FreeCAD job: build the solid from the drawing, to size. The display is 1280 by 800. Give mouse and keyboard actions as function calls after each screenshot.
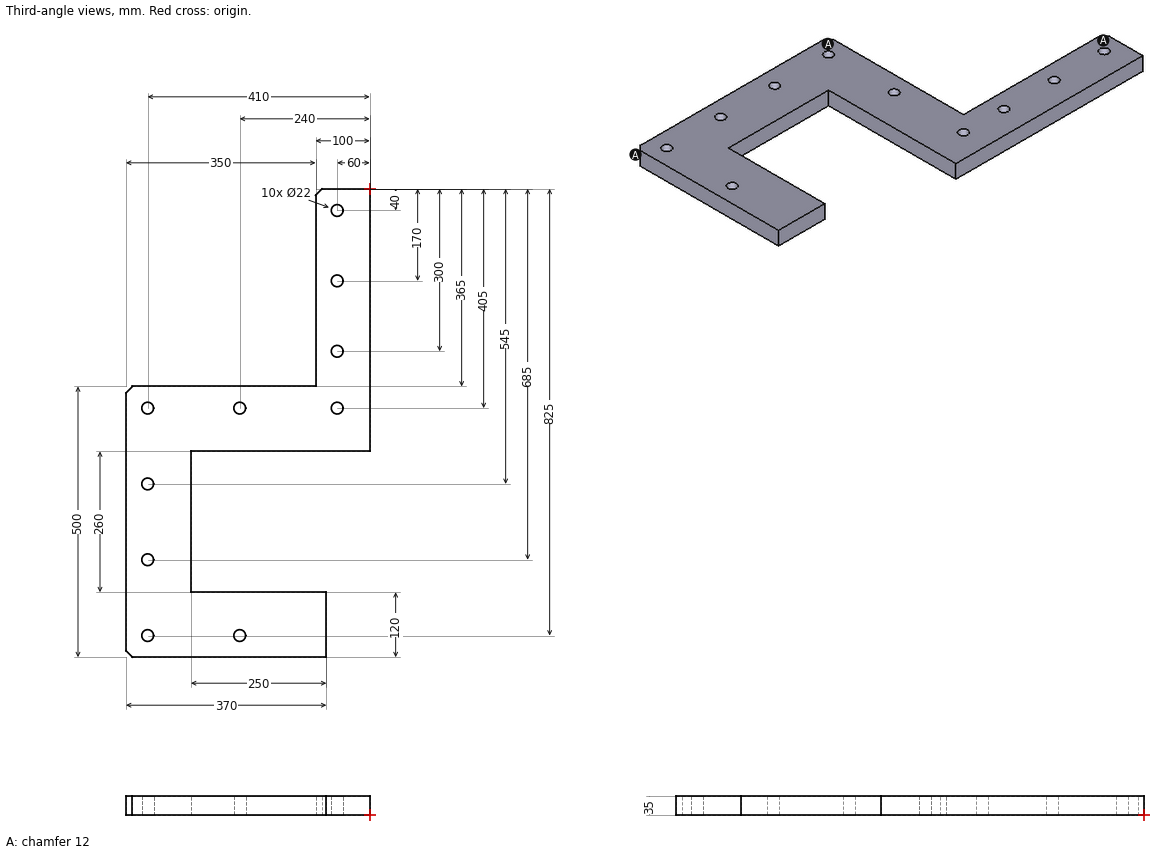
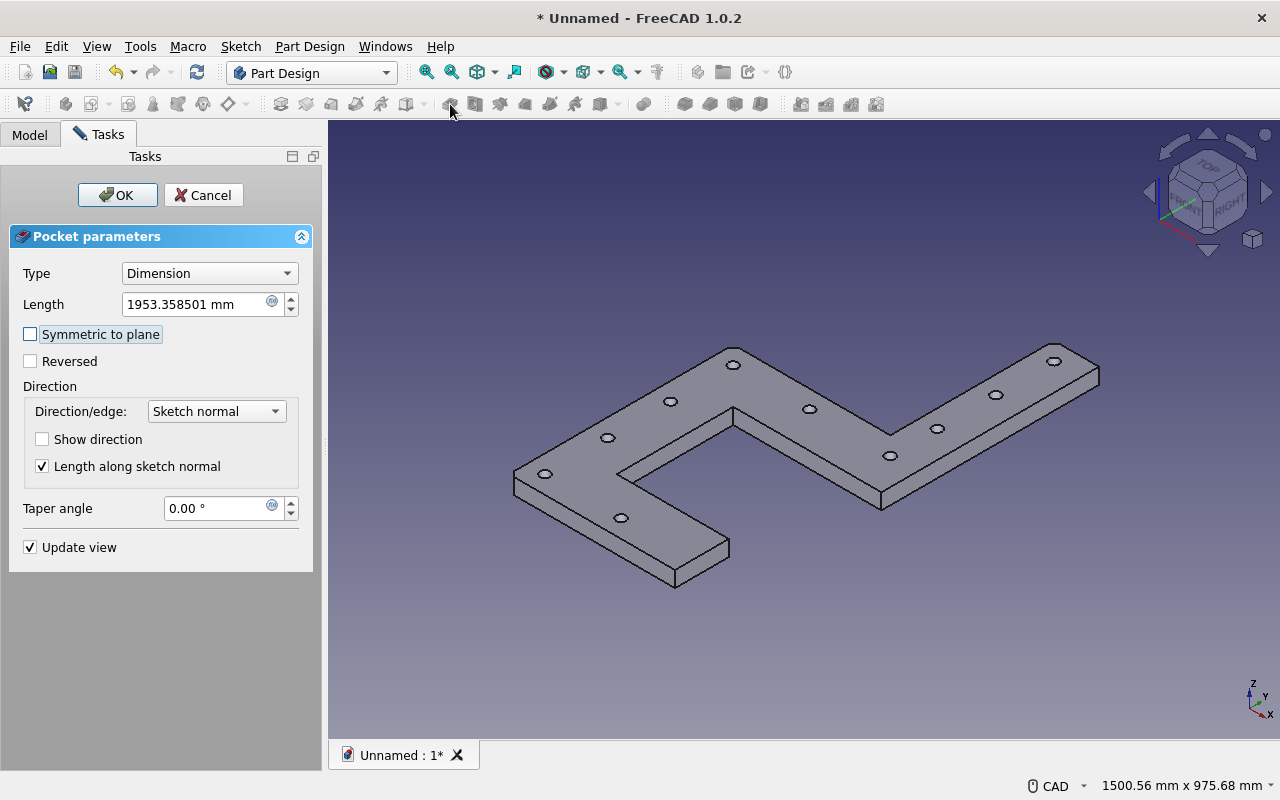
click(31, 334)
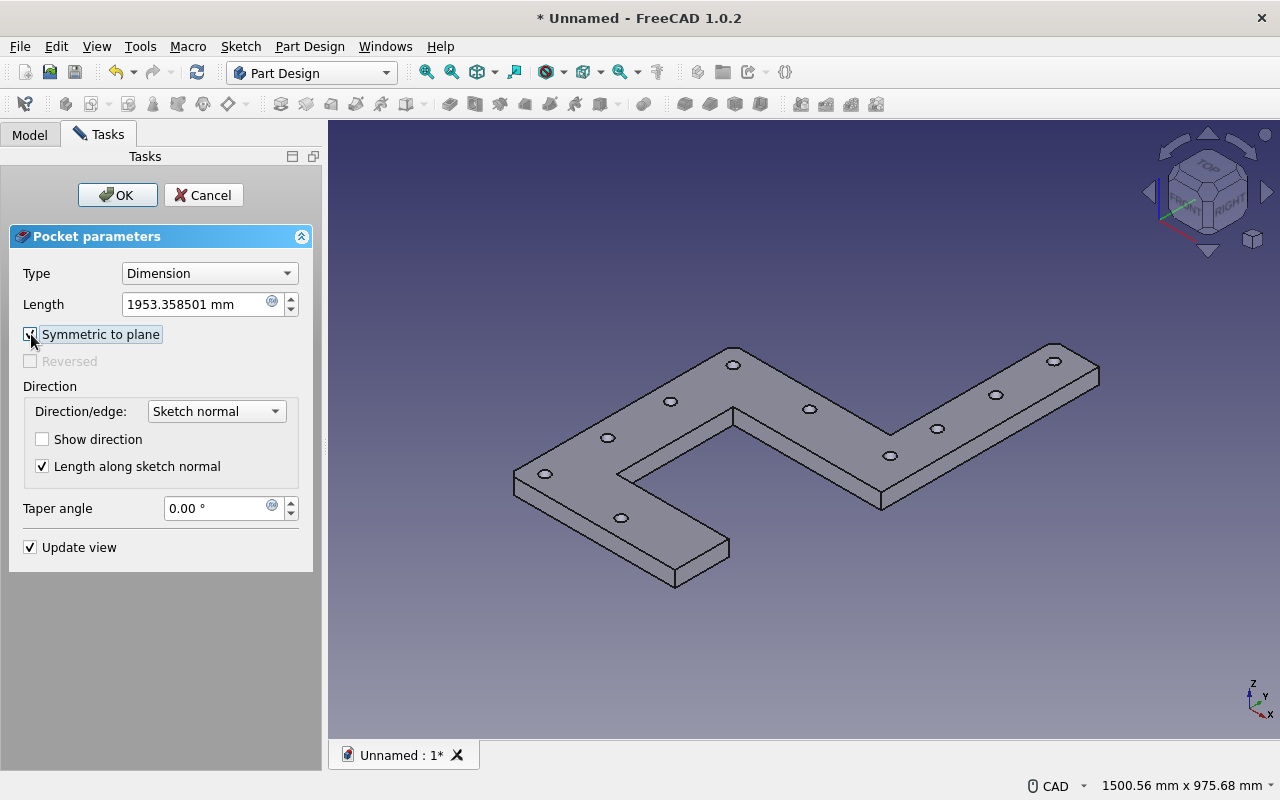
click(118, 195)